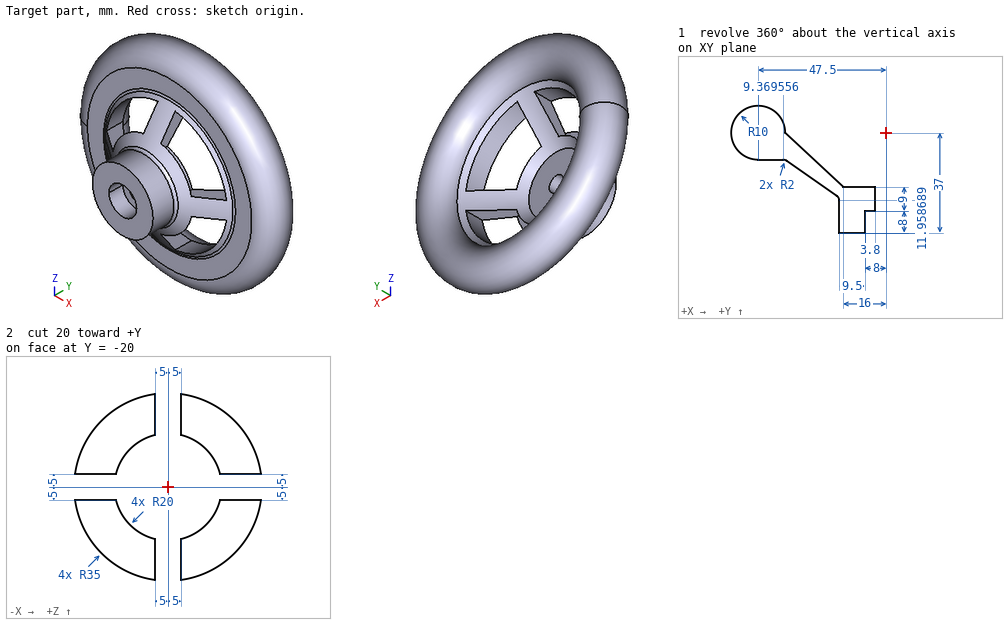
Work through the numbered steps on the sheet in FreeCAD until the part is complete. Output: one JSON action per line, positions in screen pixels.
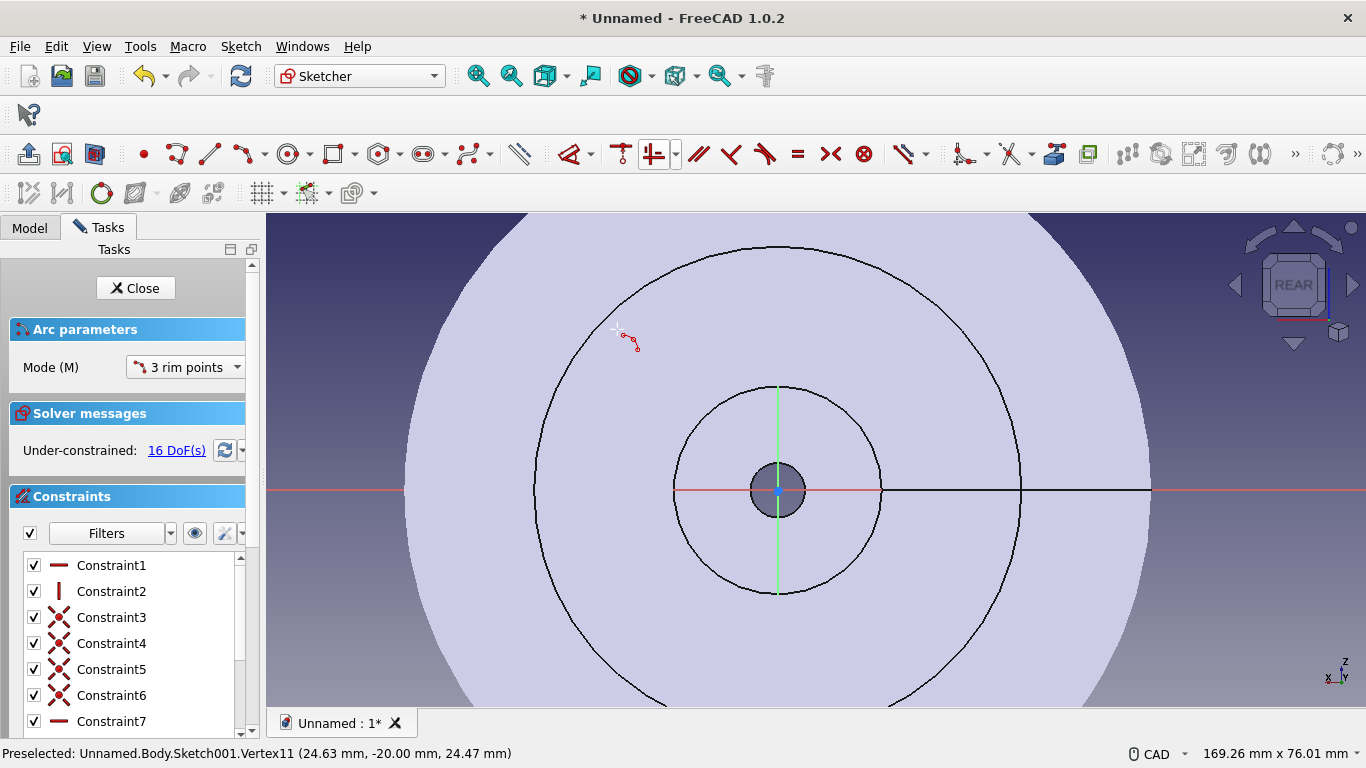
{"action": "key", "text": "g l"}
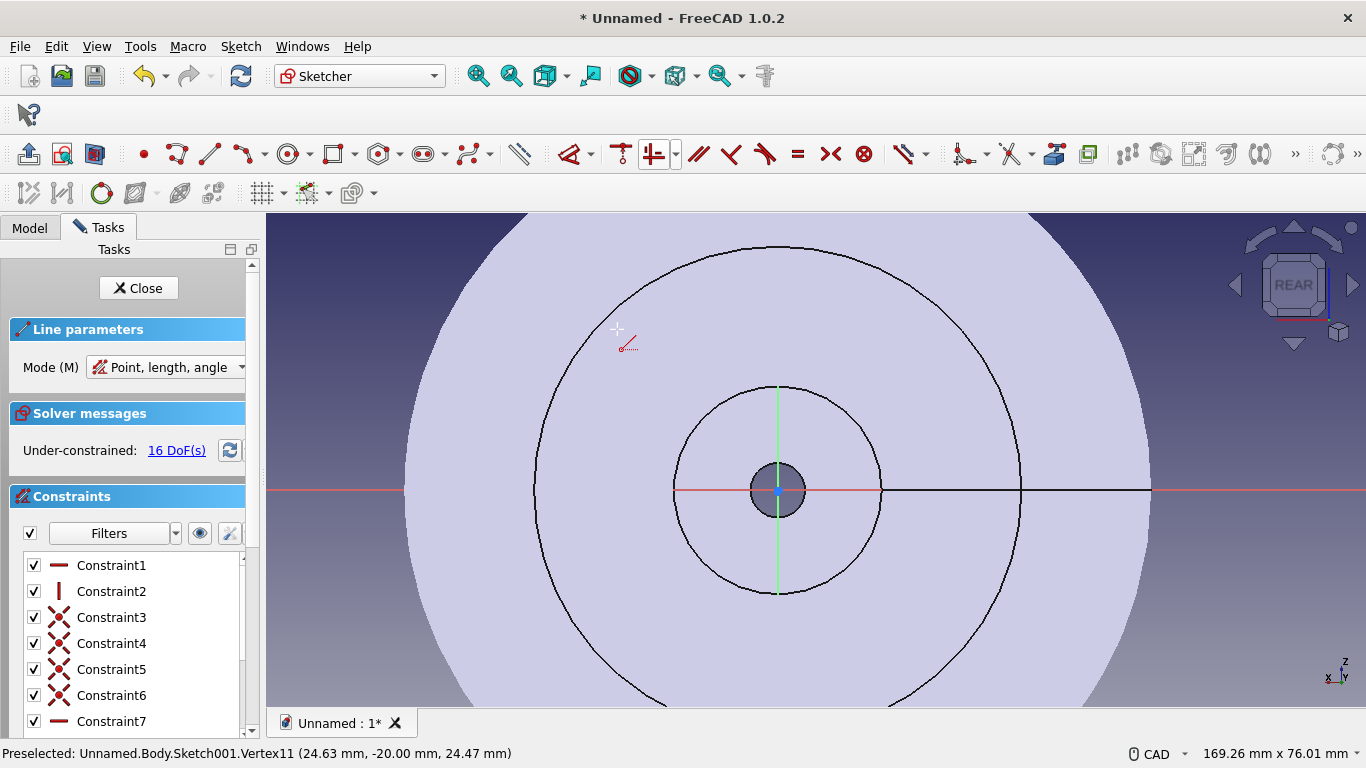
{"action": "left_click", "coordinate": [1003, 523]}
{"action": "left_click", "coordinate": [904, 523]}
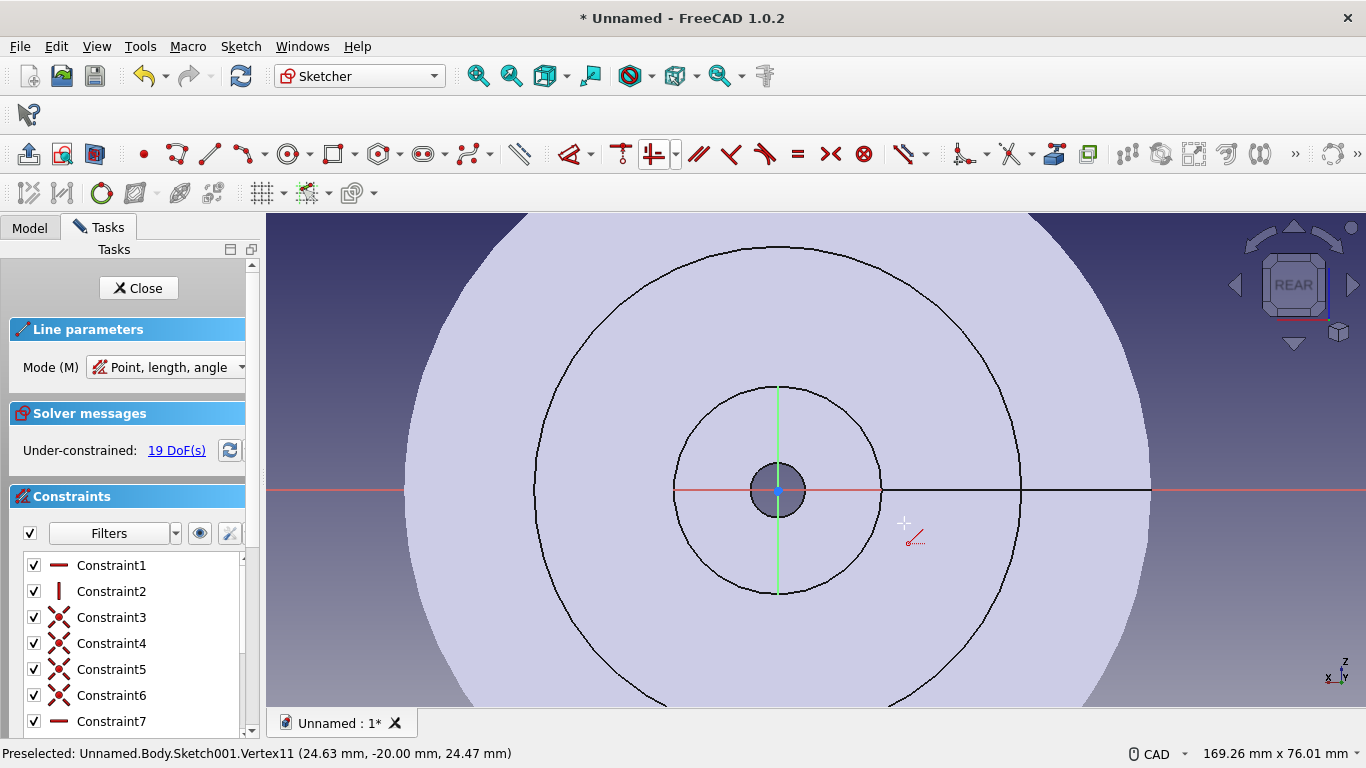
{"action": "left_click", "coordinate": [810, 616]}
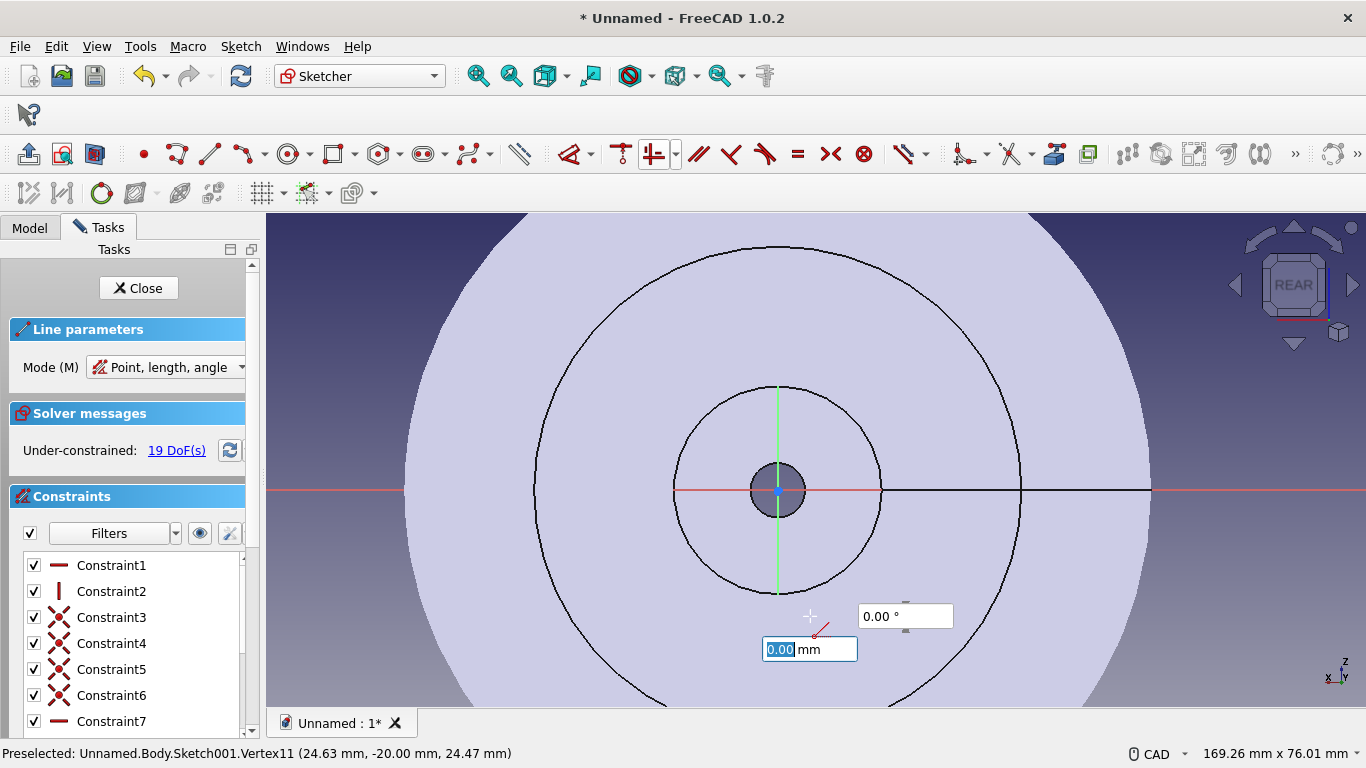
{"action": "scroll", "coordinate": [686, 398], "scroll_direction": "down", "scroll_amount": 2}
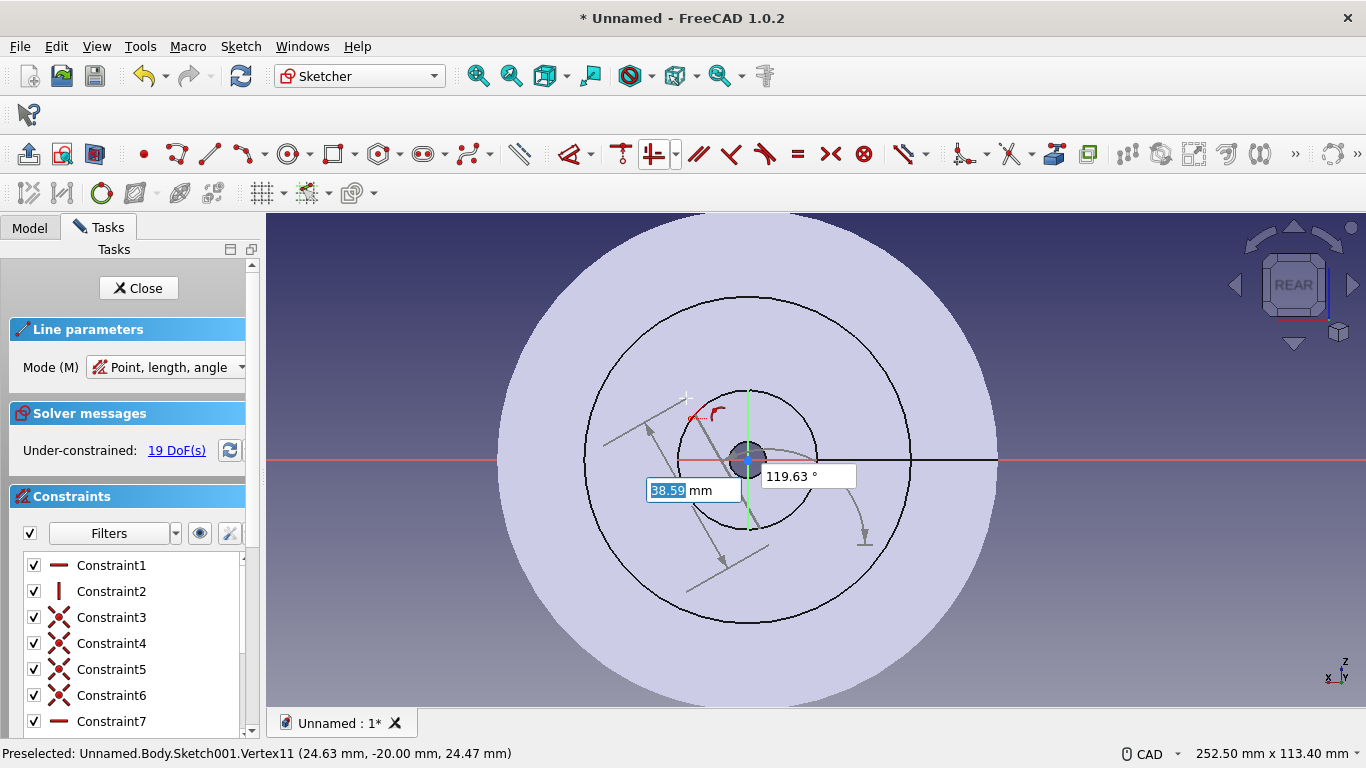
{"action": "left_click", "coordinate": [769, 611]}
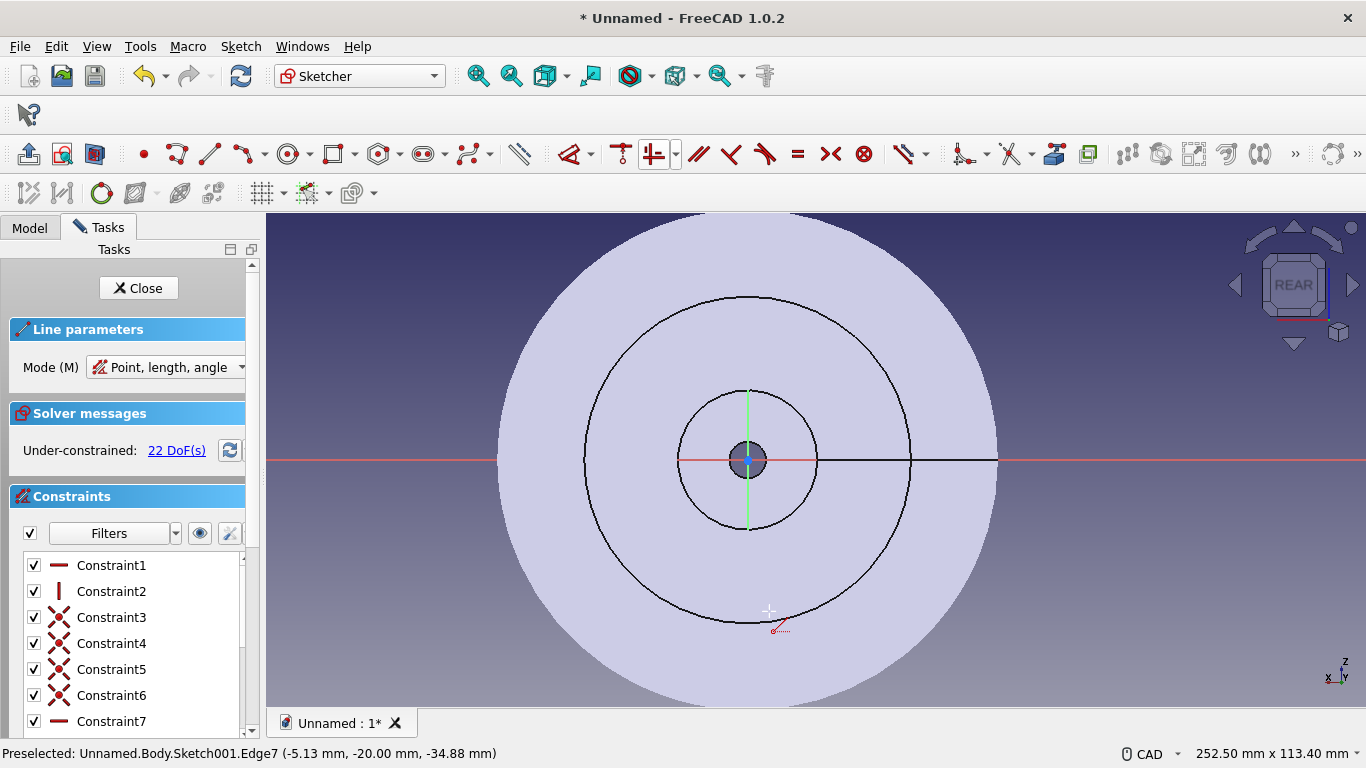
{"action": "left_click", "coordinate": [242, 154]}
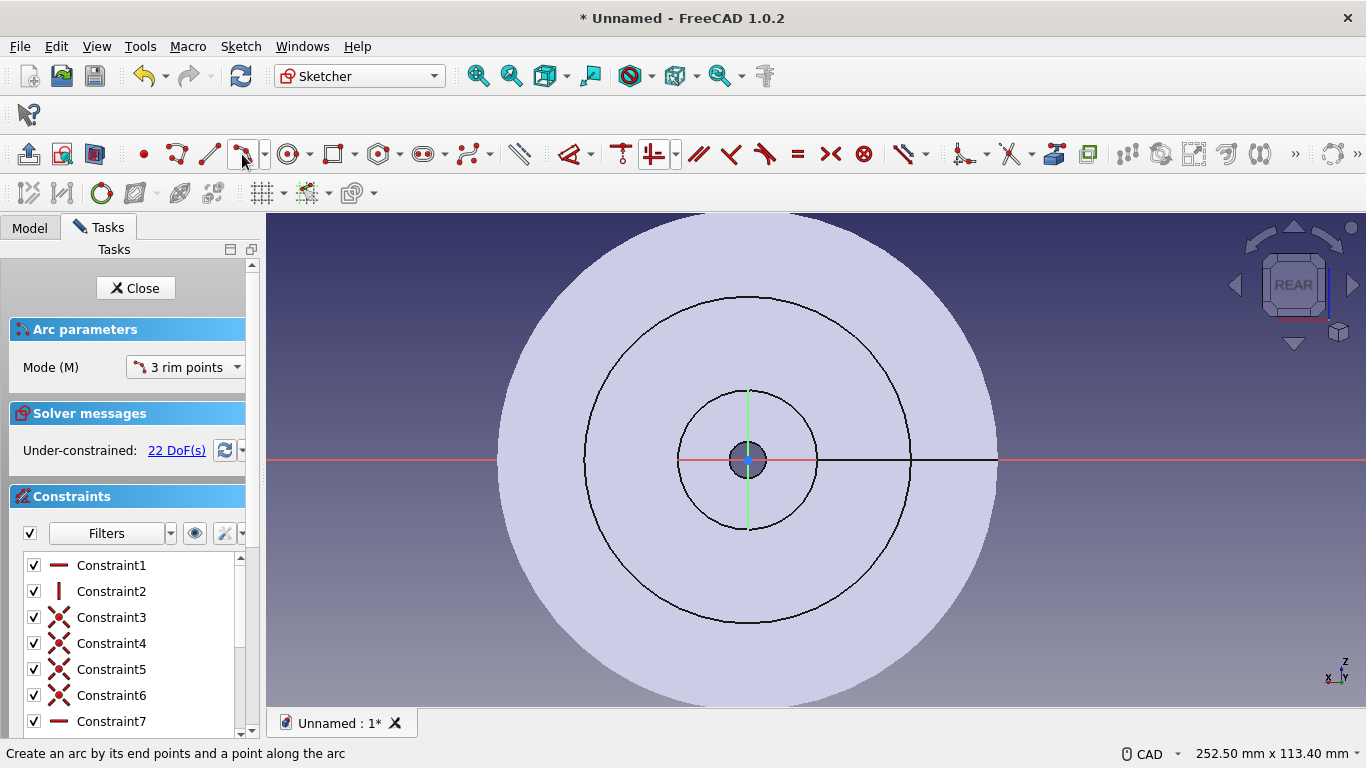
{"action": "left_click", "coordinate": [832, 483]}
{"action": "left_click", "coordinate": [769, 545]}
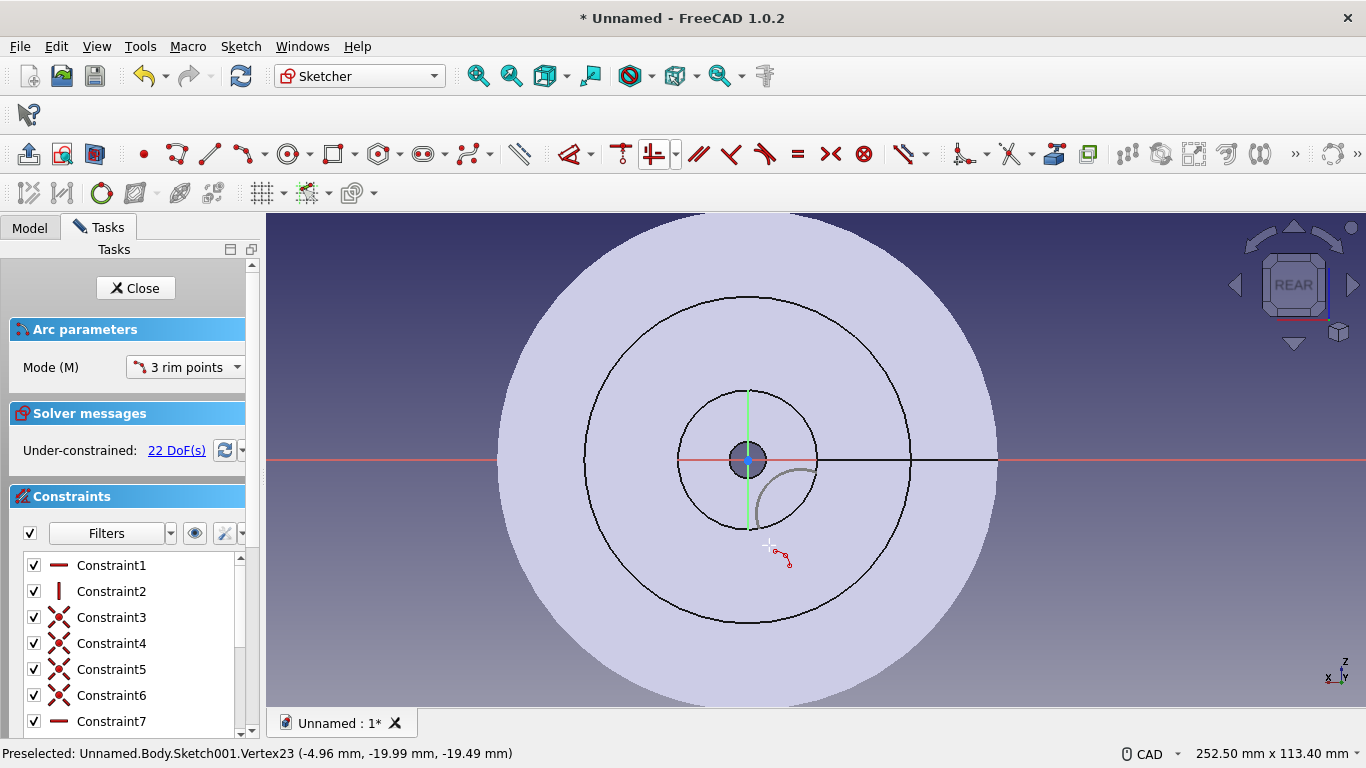
{"action": "scroll", "coordinate": [809, 522], "scroll_direction": "up", "scroll_amount": 2}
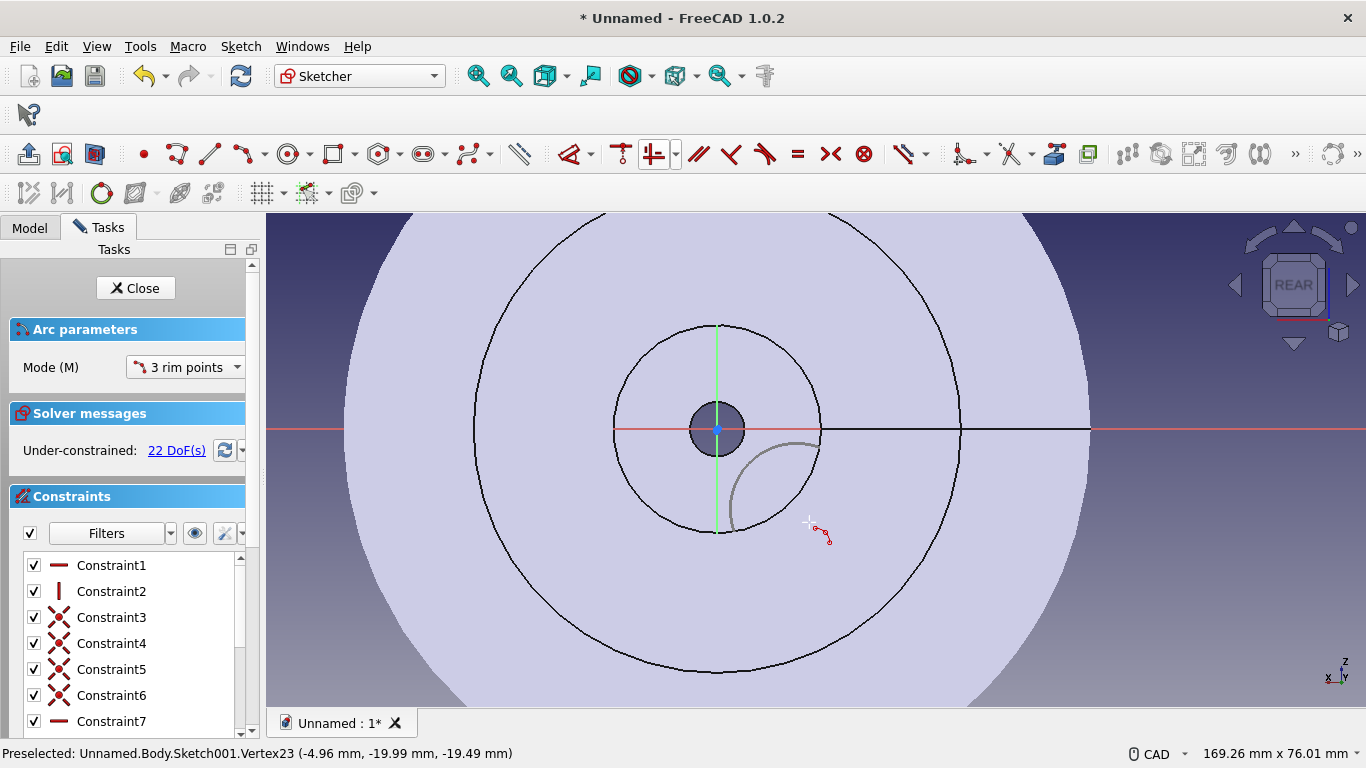
{"action": "left_click", "coordinate": [809, 521]}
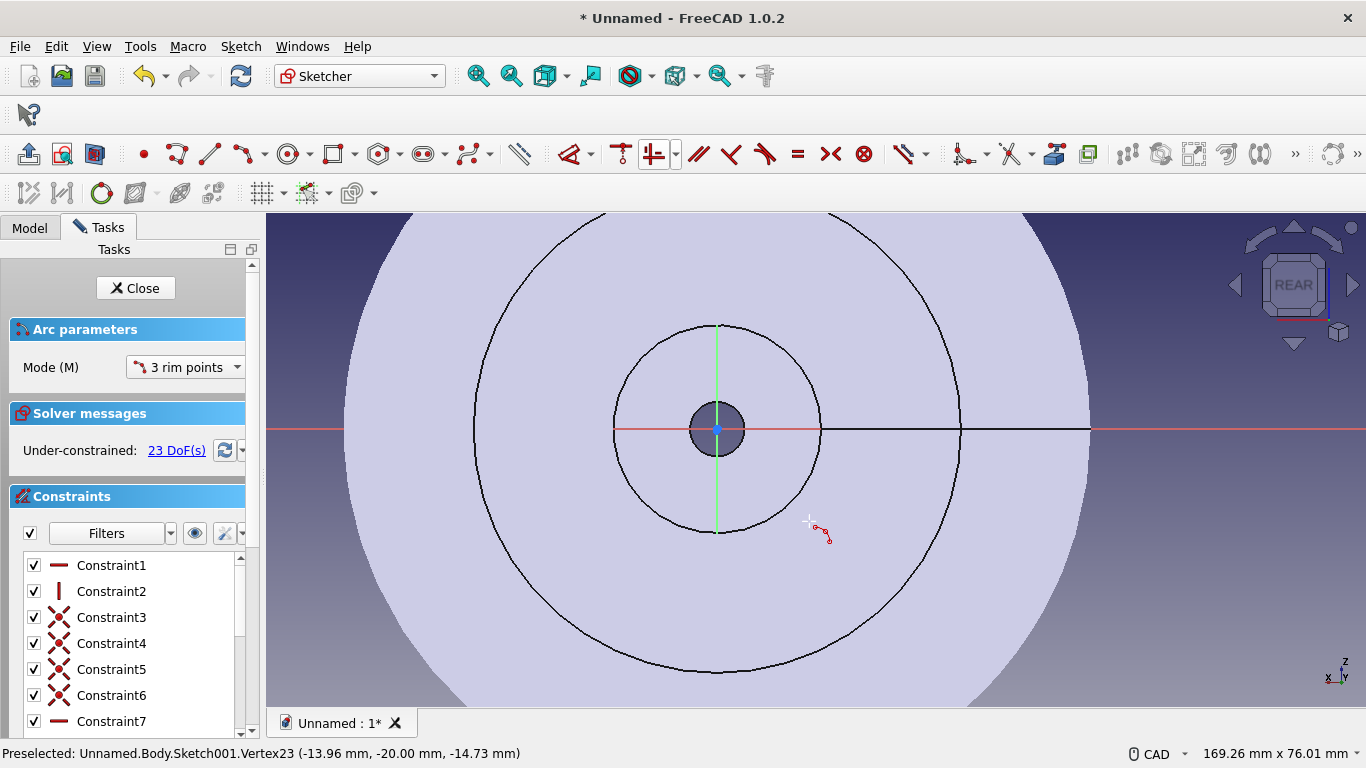
{"action": "left_click", "coordinate": [749, 656]}
{"action": "left_click", "coordinate": [942, 463]}
{"action": "left_click", "coordinate": [878, 590]}